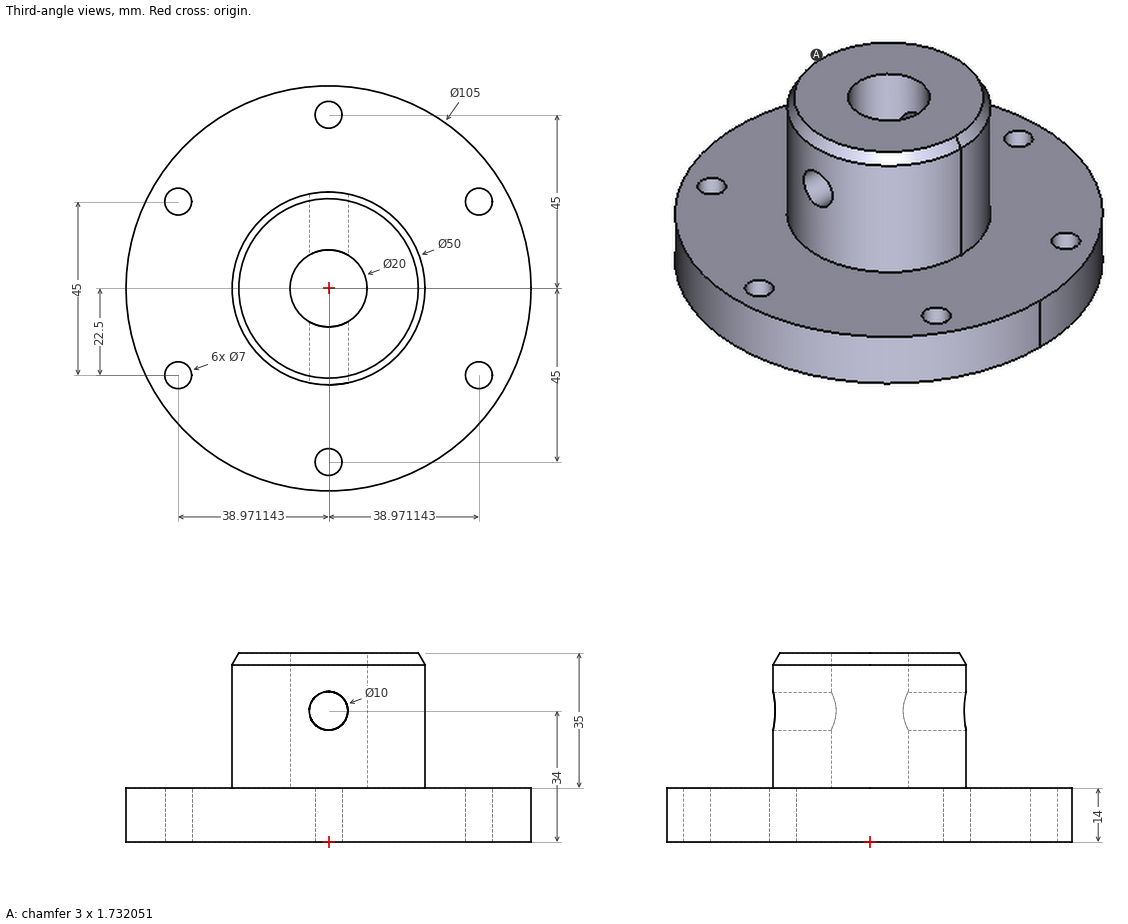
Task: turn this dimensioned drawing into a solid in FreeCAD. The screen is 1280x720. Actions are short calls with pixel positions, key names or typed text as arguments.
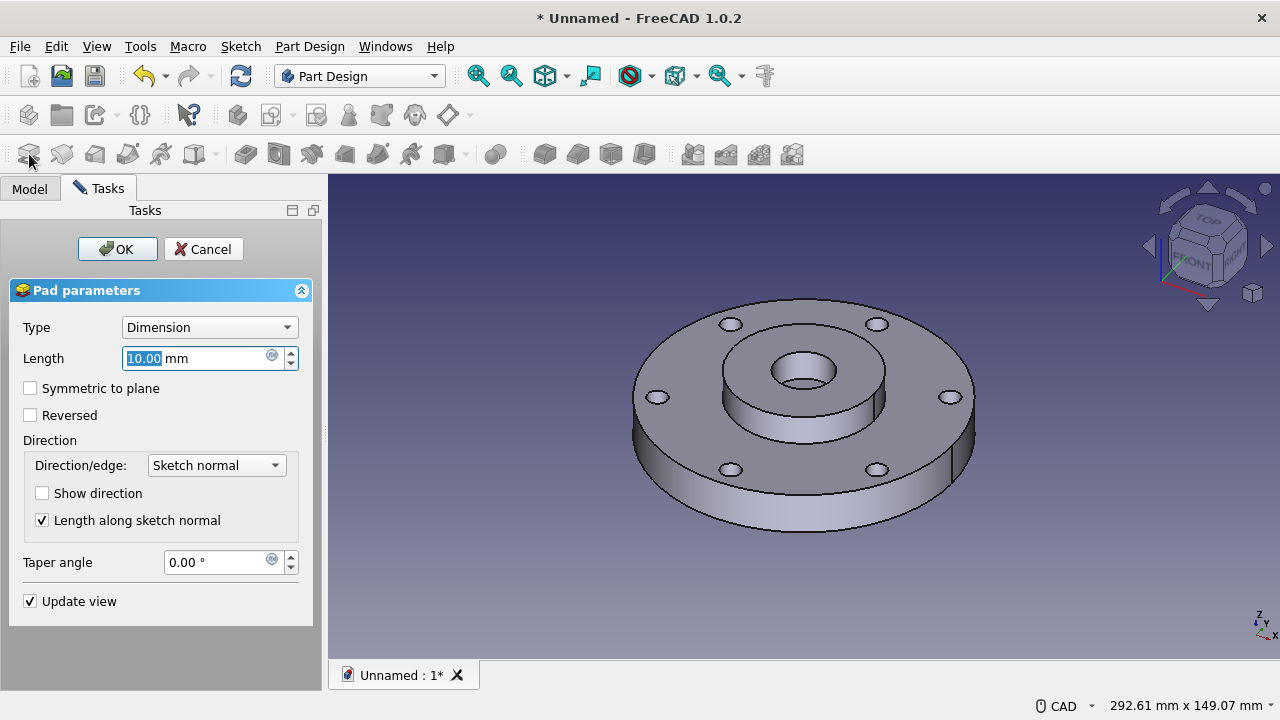
text(35)
key(Tab)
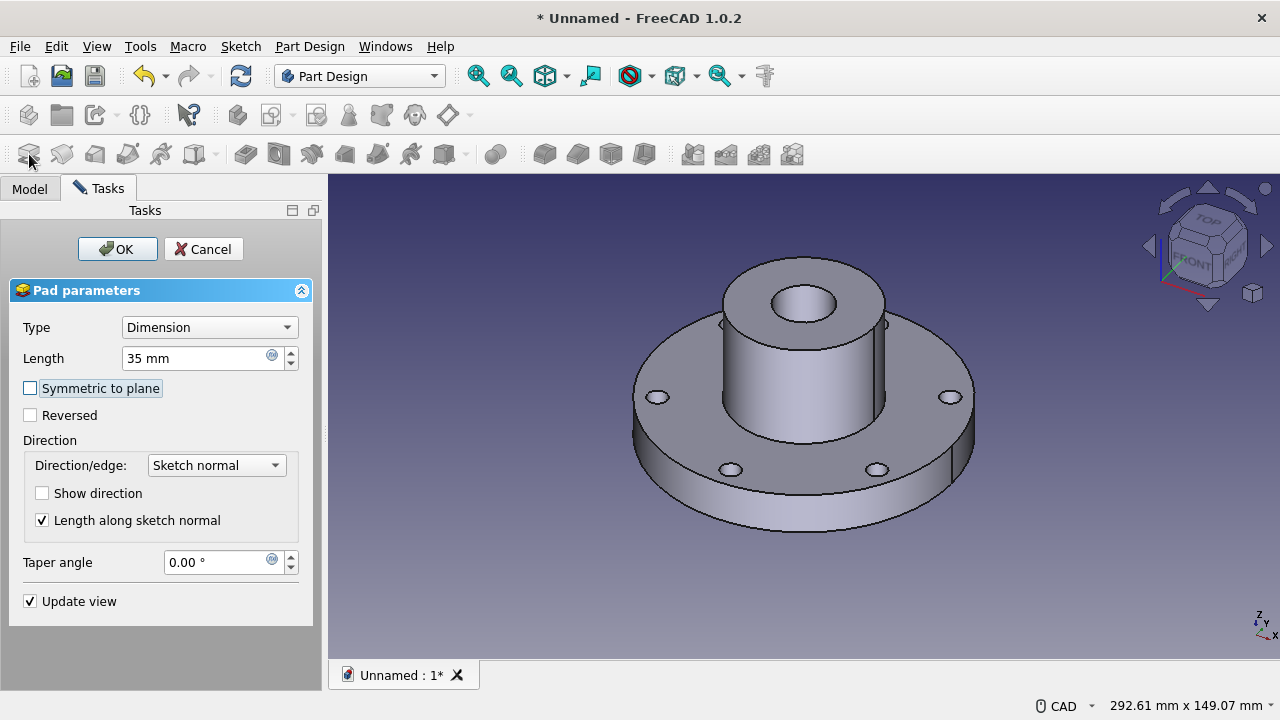
click(118, 249)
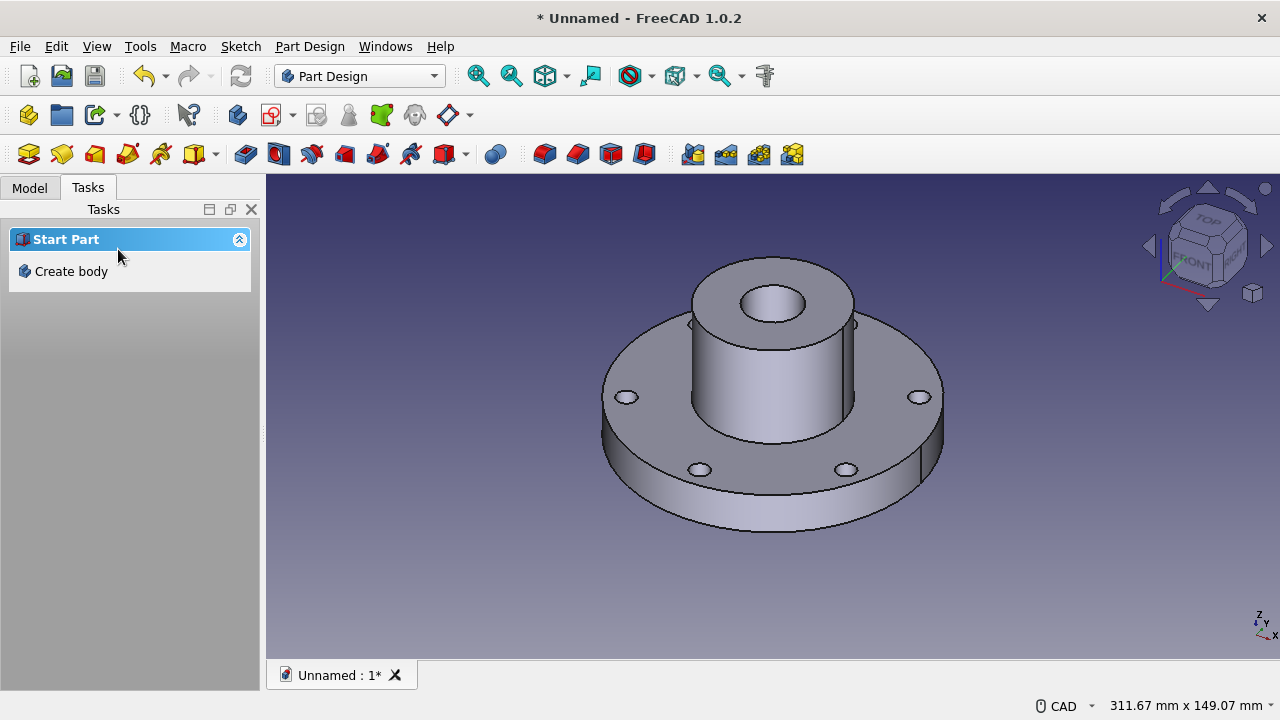
click(479, 76)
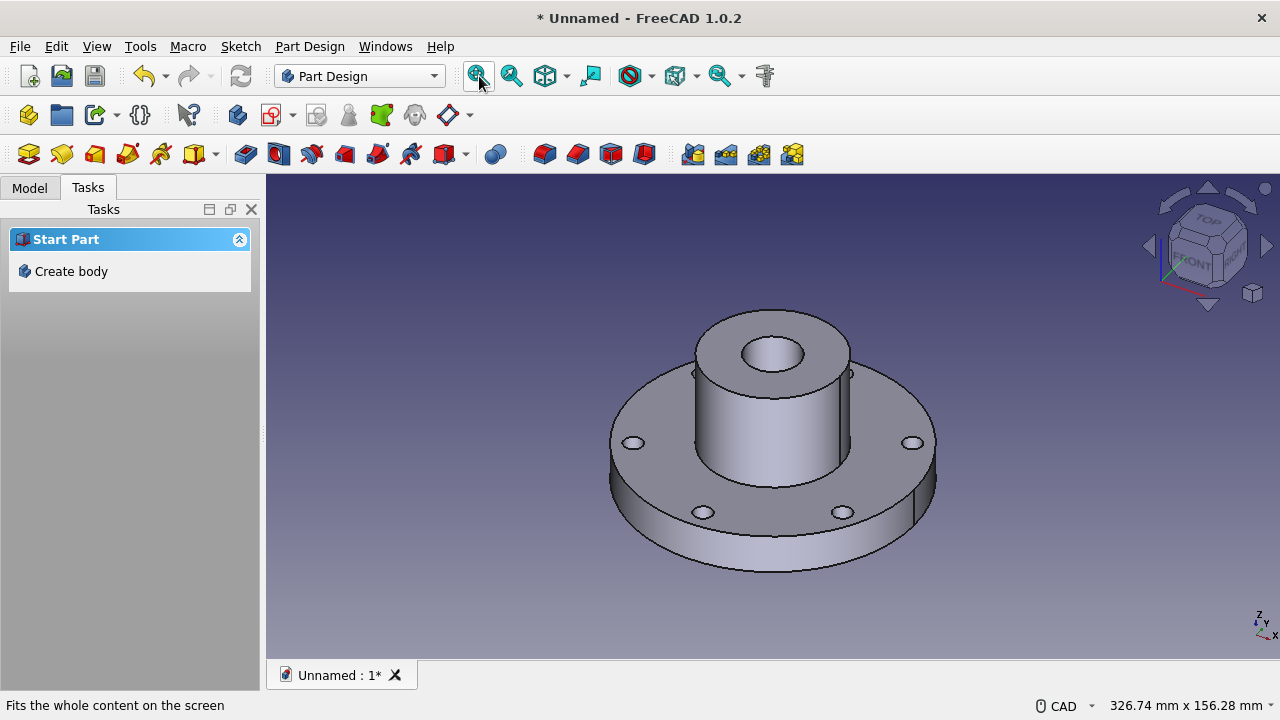
click(270, 116)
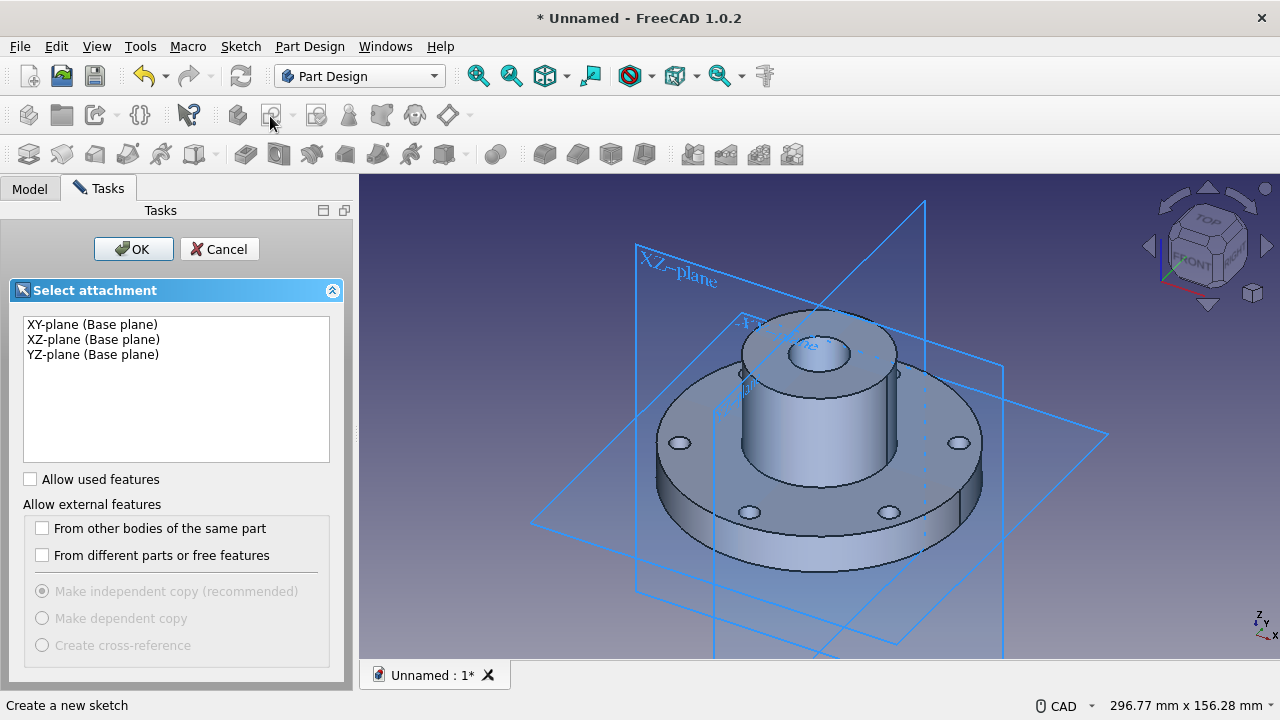
click(84, 340)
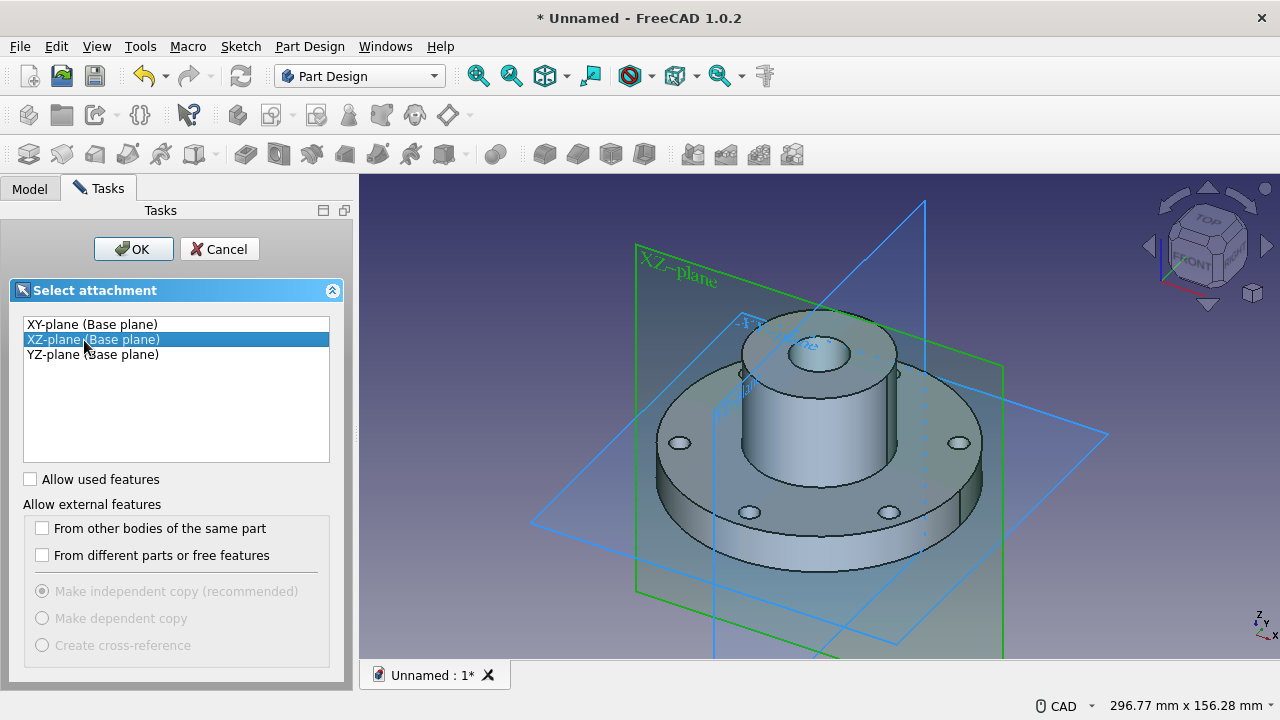
click(134, 249)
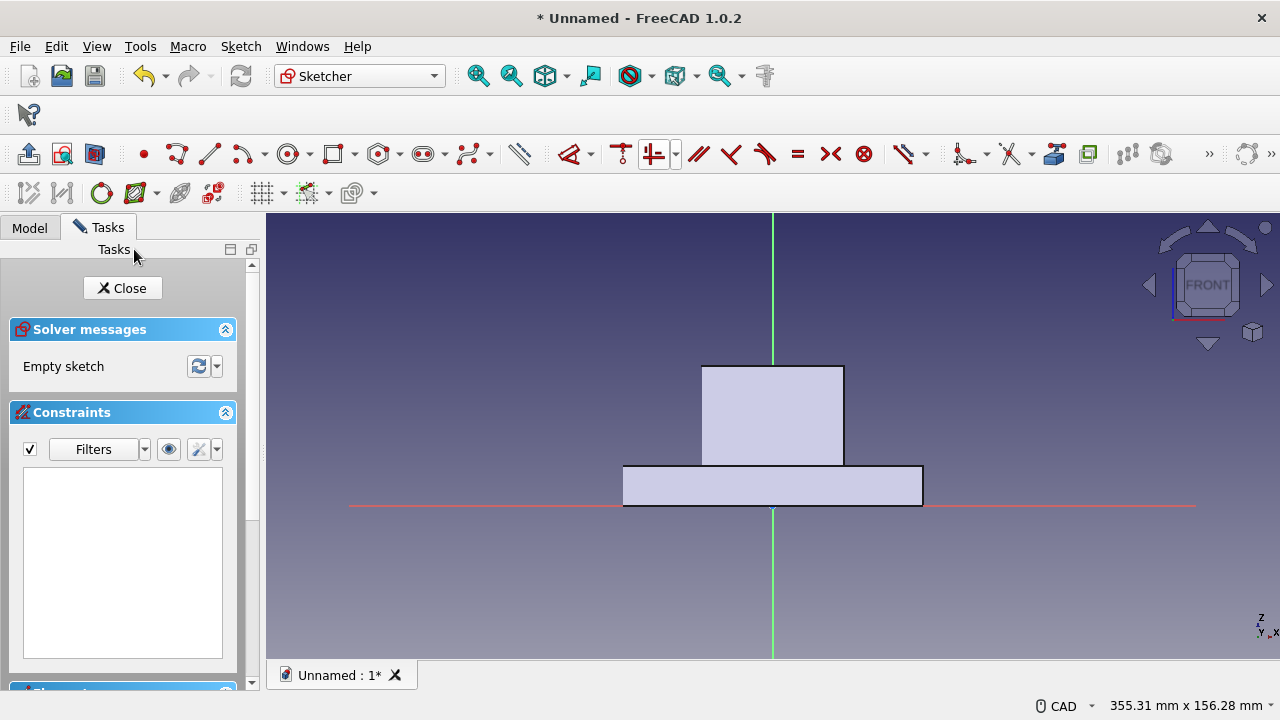
click(95, 154)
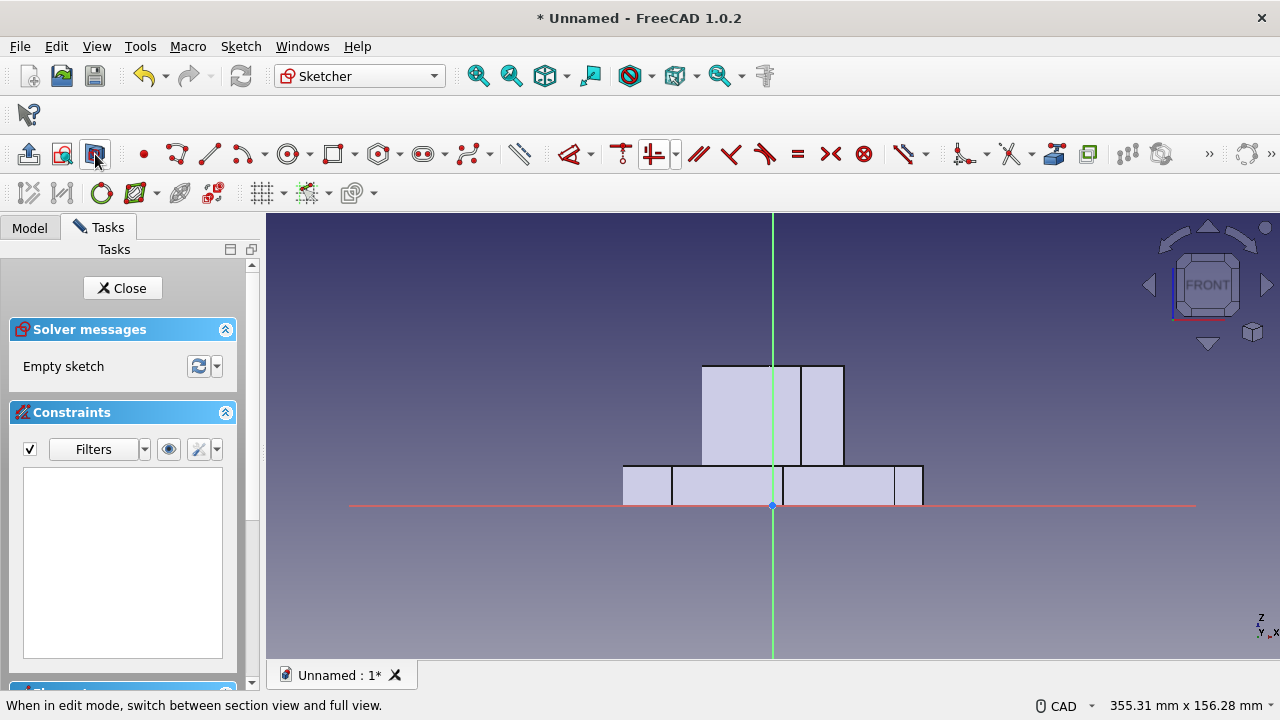
scroll(781, 406, up, 11)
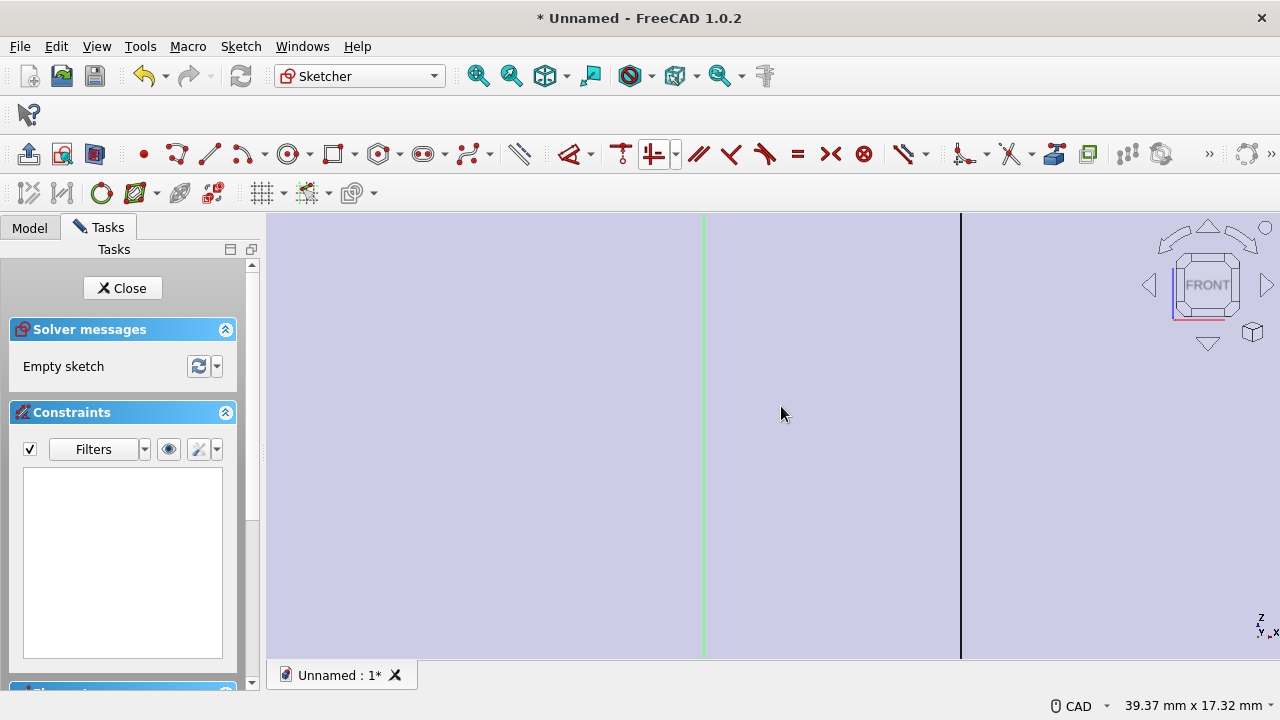
click(288, 154)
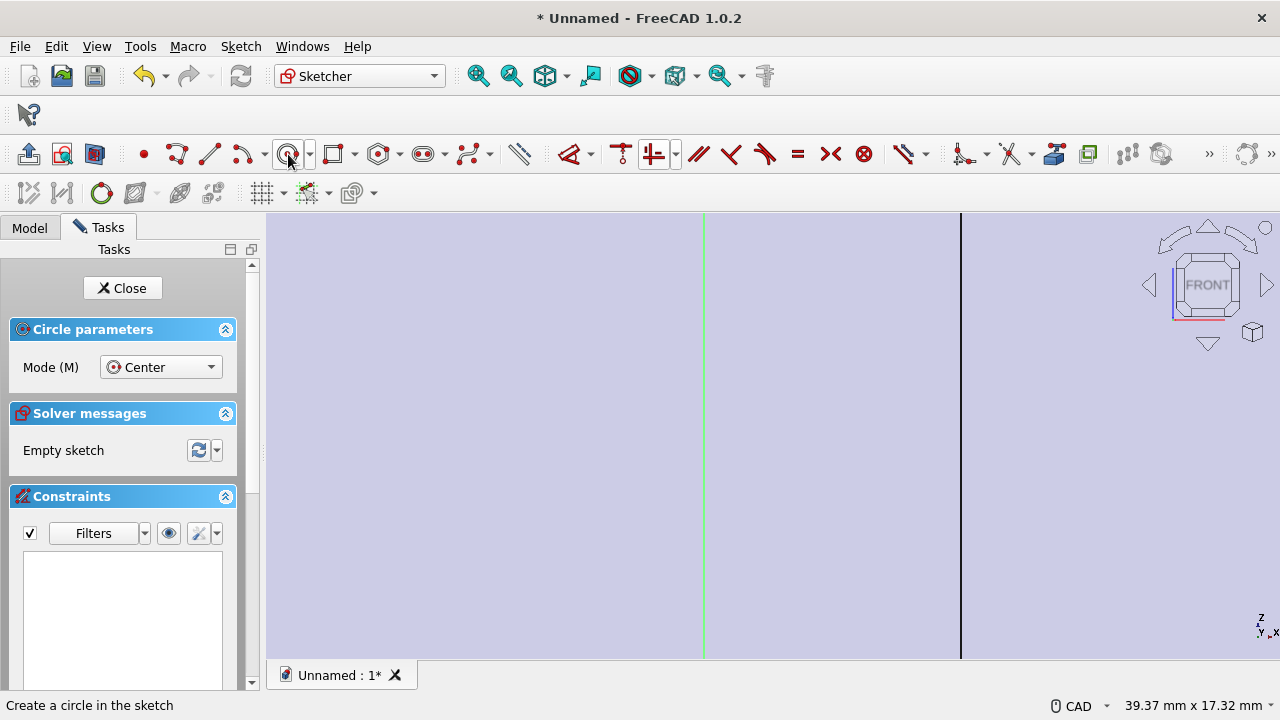
click(704, 429)
click(795, 338)
key(Escape)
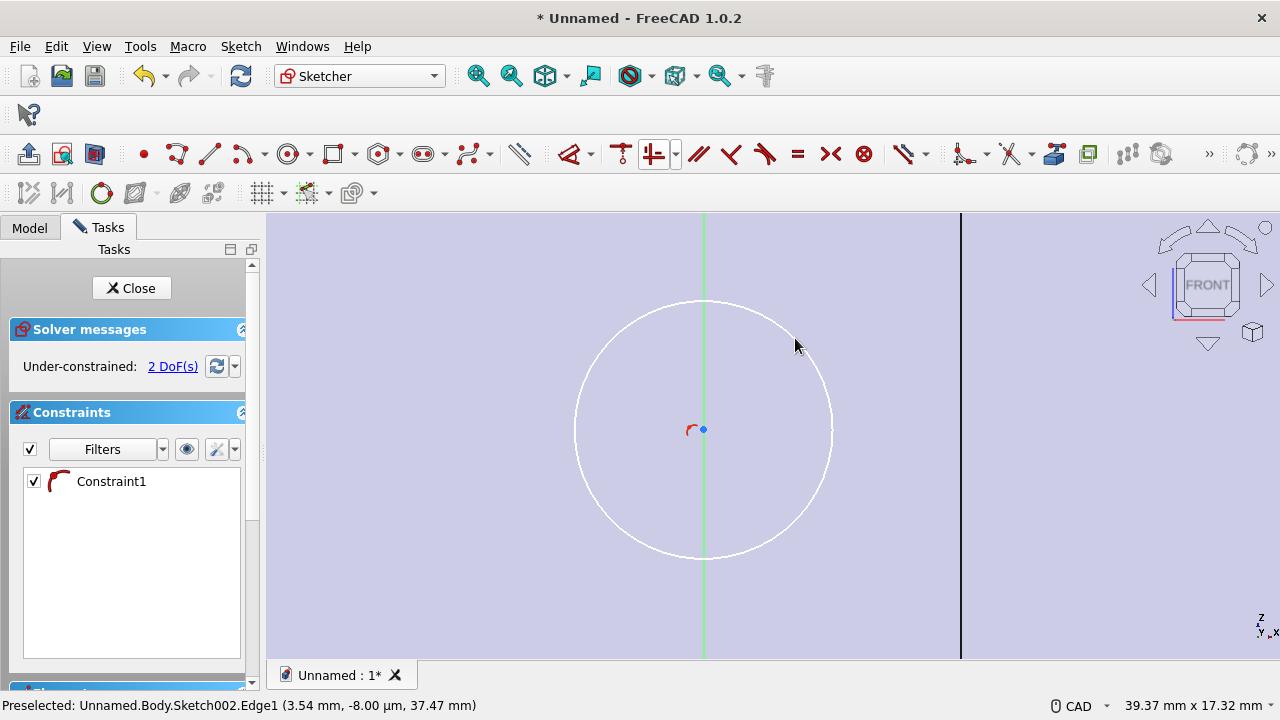
click(568, 154)